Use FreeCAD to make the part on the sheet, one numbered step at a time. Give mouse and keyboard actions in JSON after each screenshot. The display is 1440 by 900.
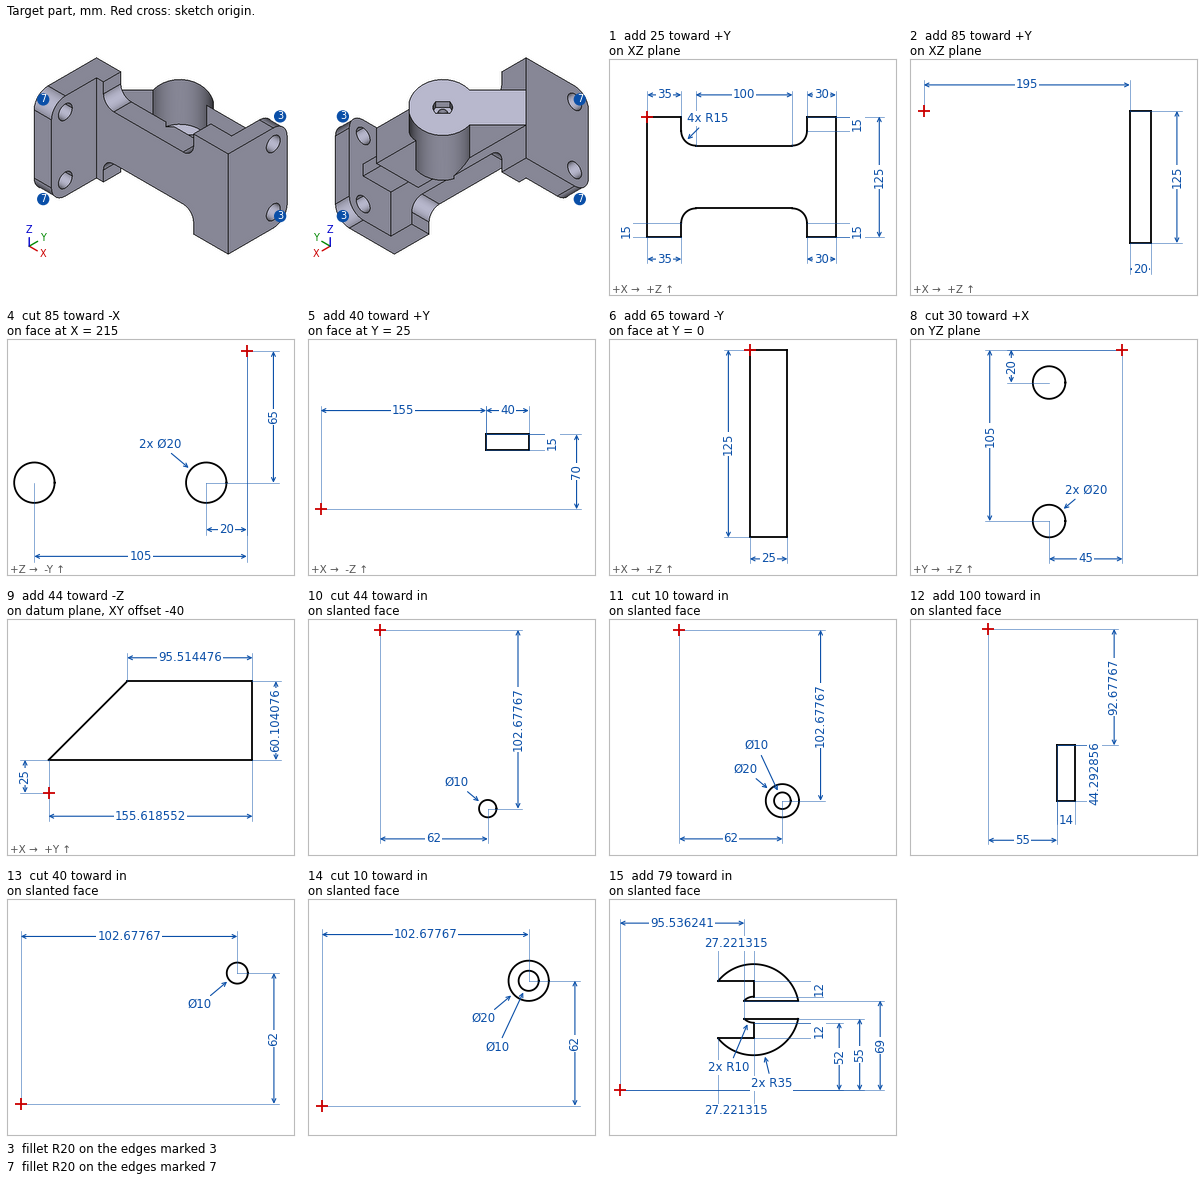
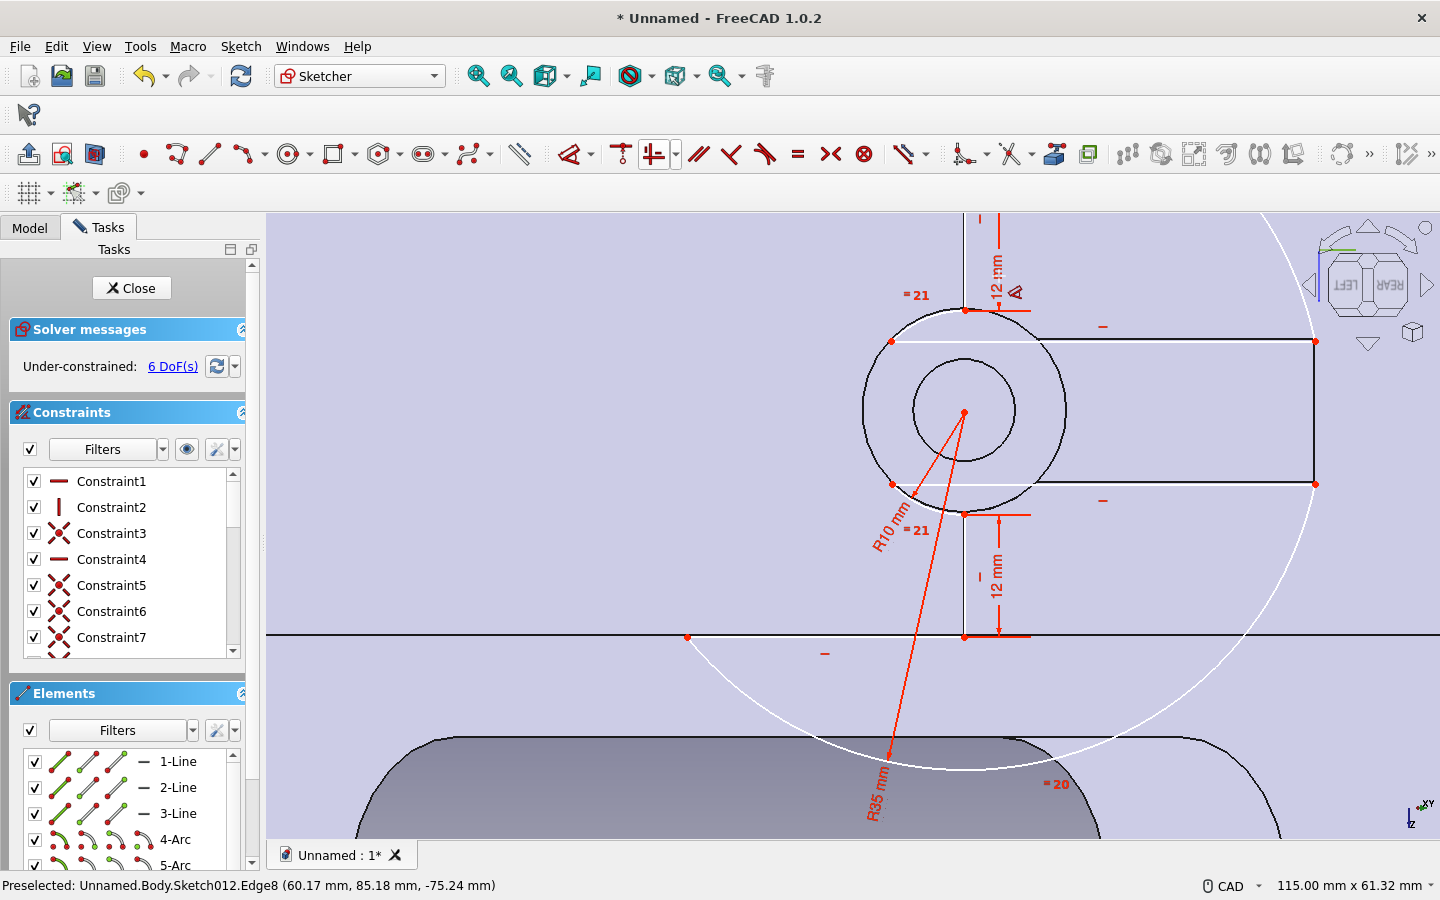
{"action": "scroll", "coordinate": [923, 504], "scroll_direction": "down", "scroll_amount": 4}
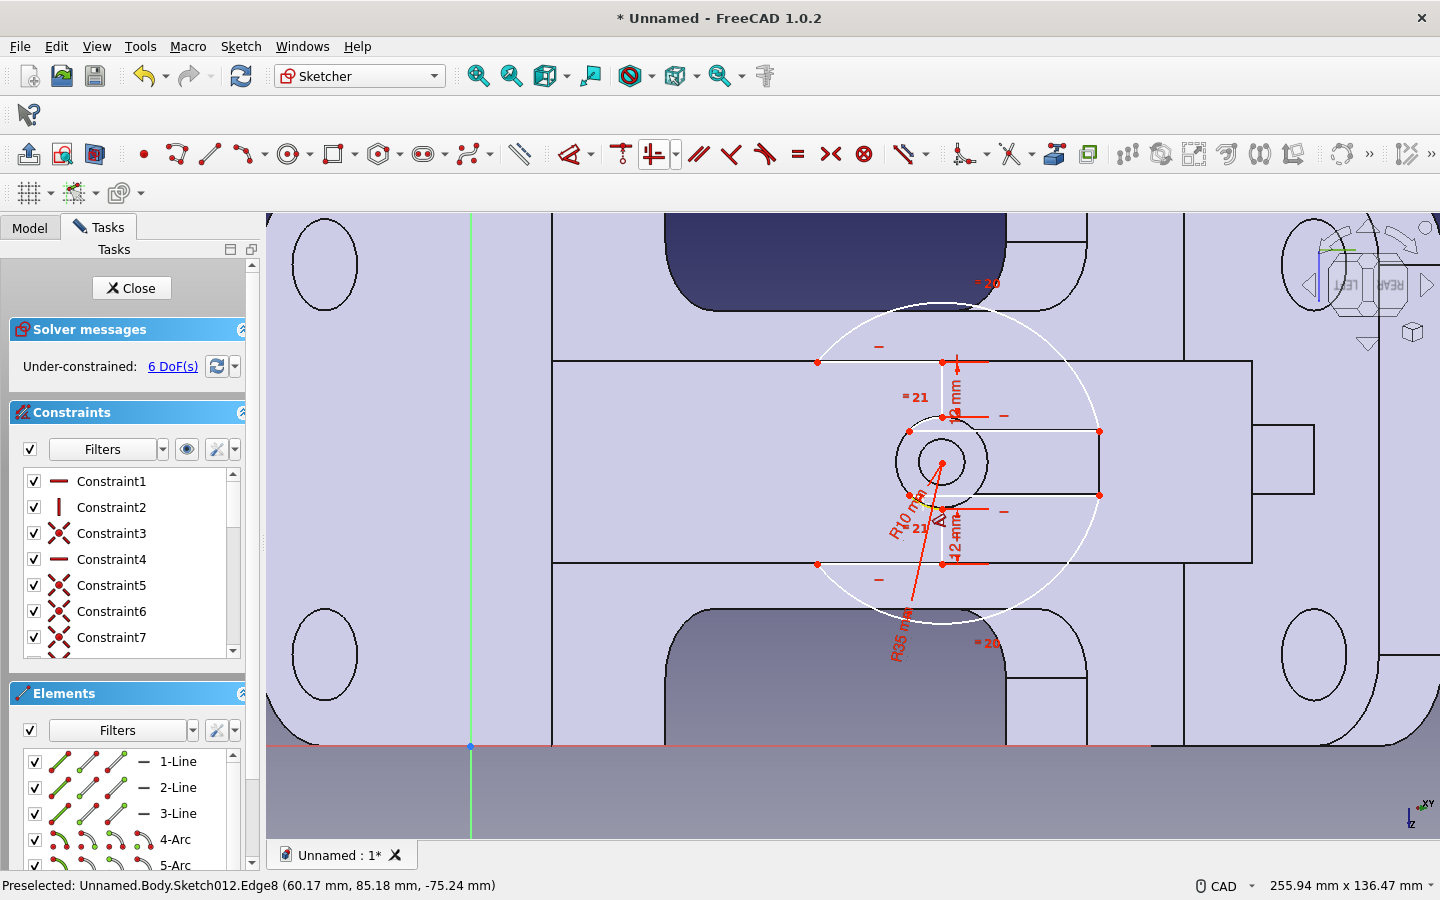
{"action": "left_click", "coordinate": [1099, 496]}
{"action": "left_click", "coordinate": [1133, 621]}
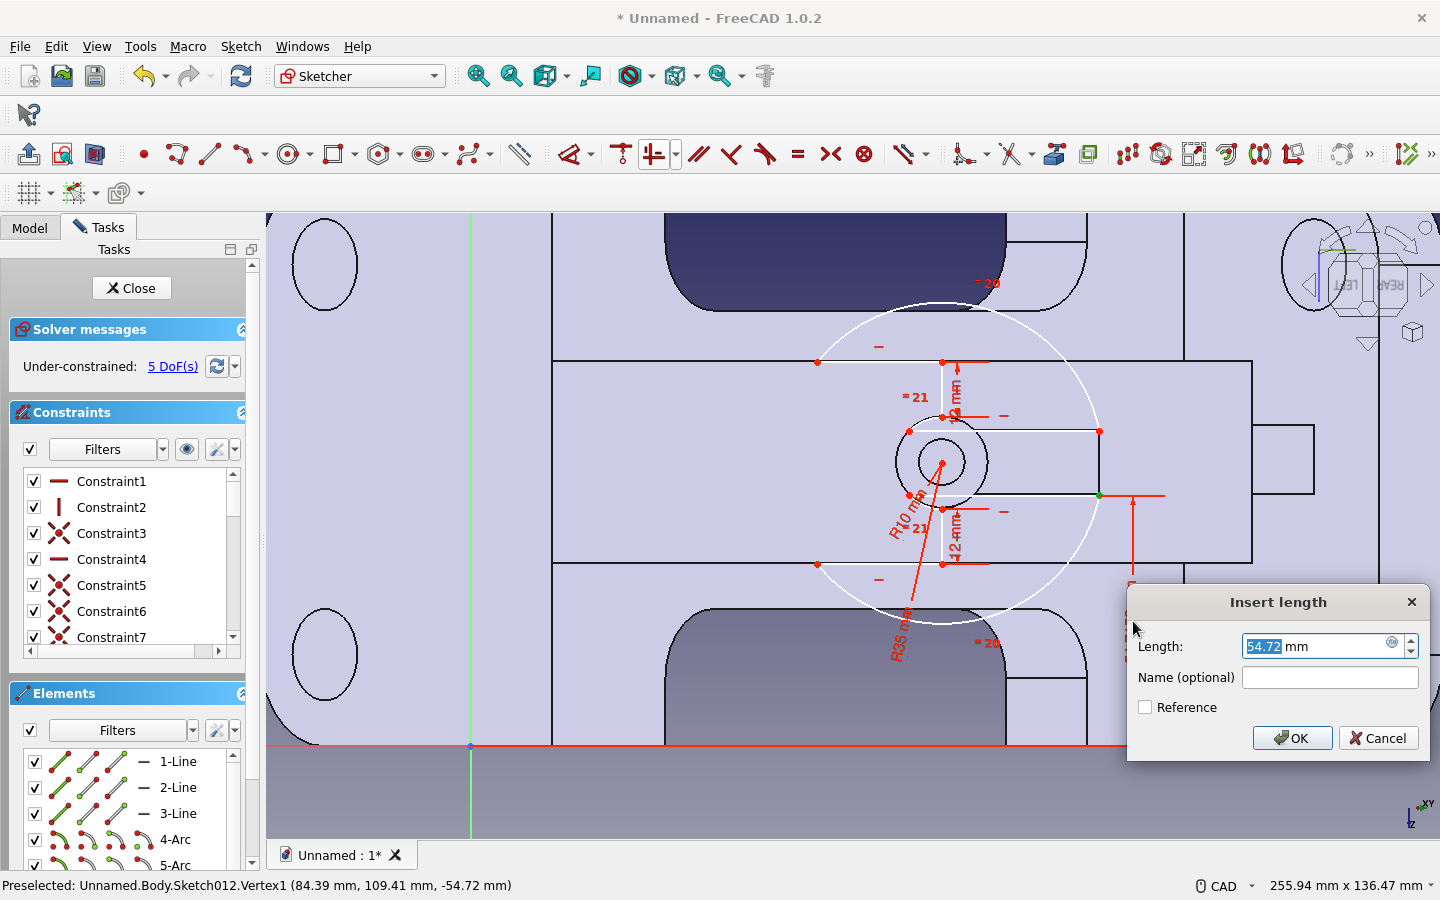
{"action": "type", "text": "55"}
{"action": "key", "text": "Return"}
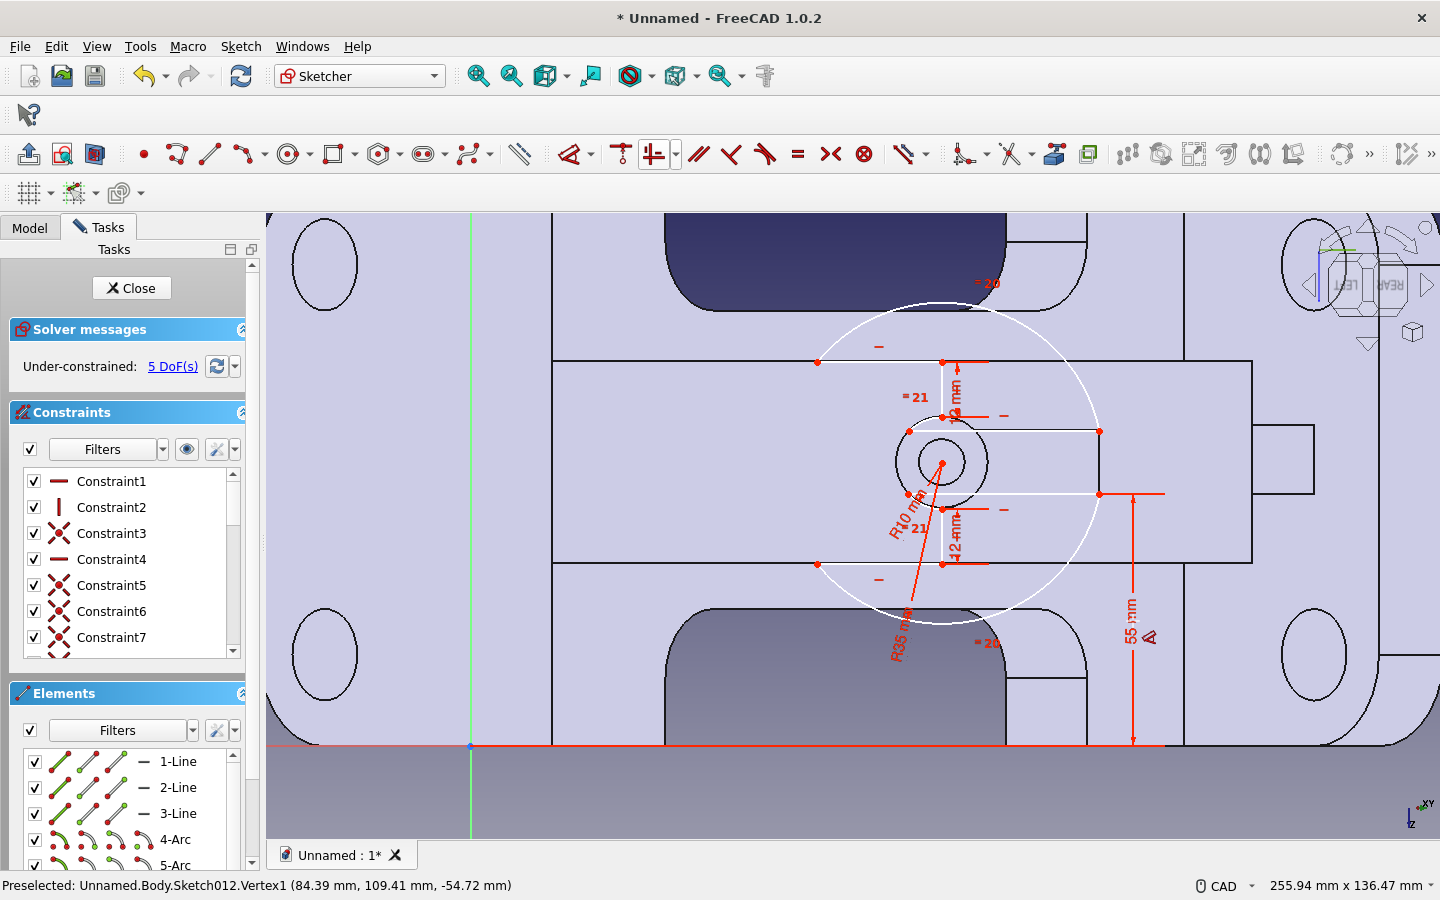
{"action": "left_click", "coordinate": [942, 509]}
{"action": "left_click", "coordinate": [437, 628]}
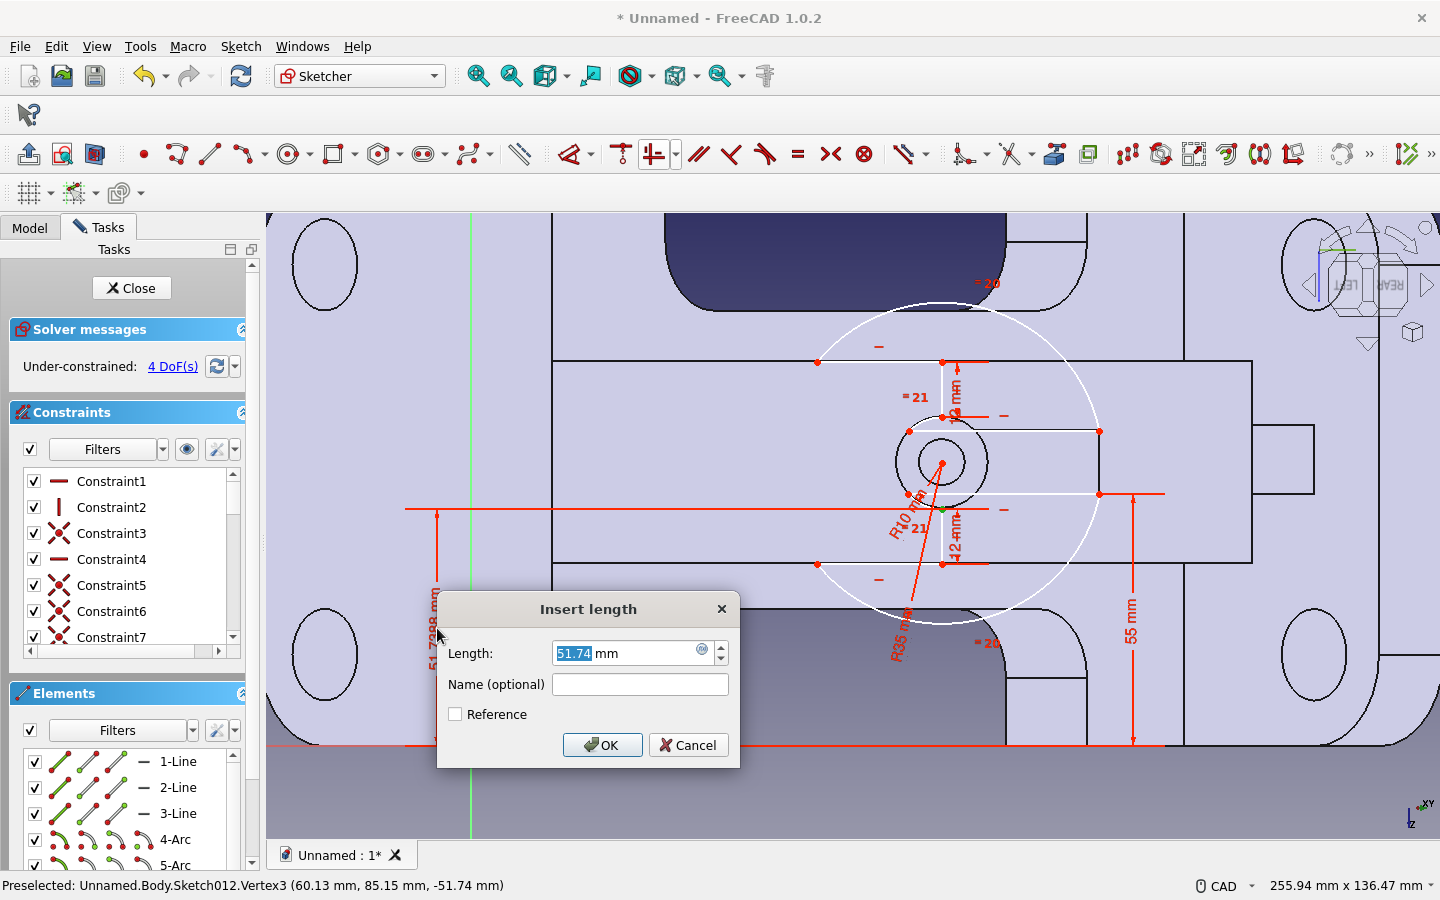
{"action": "type", "text": "52"}
{"action": "key", "text": "Return"}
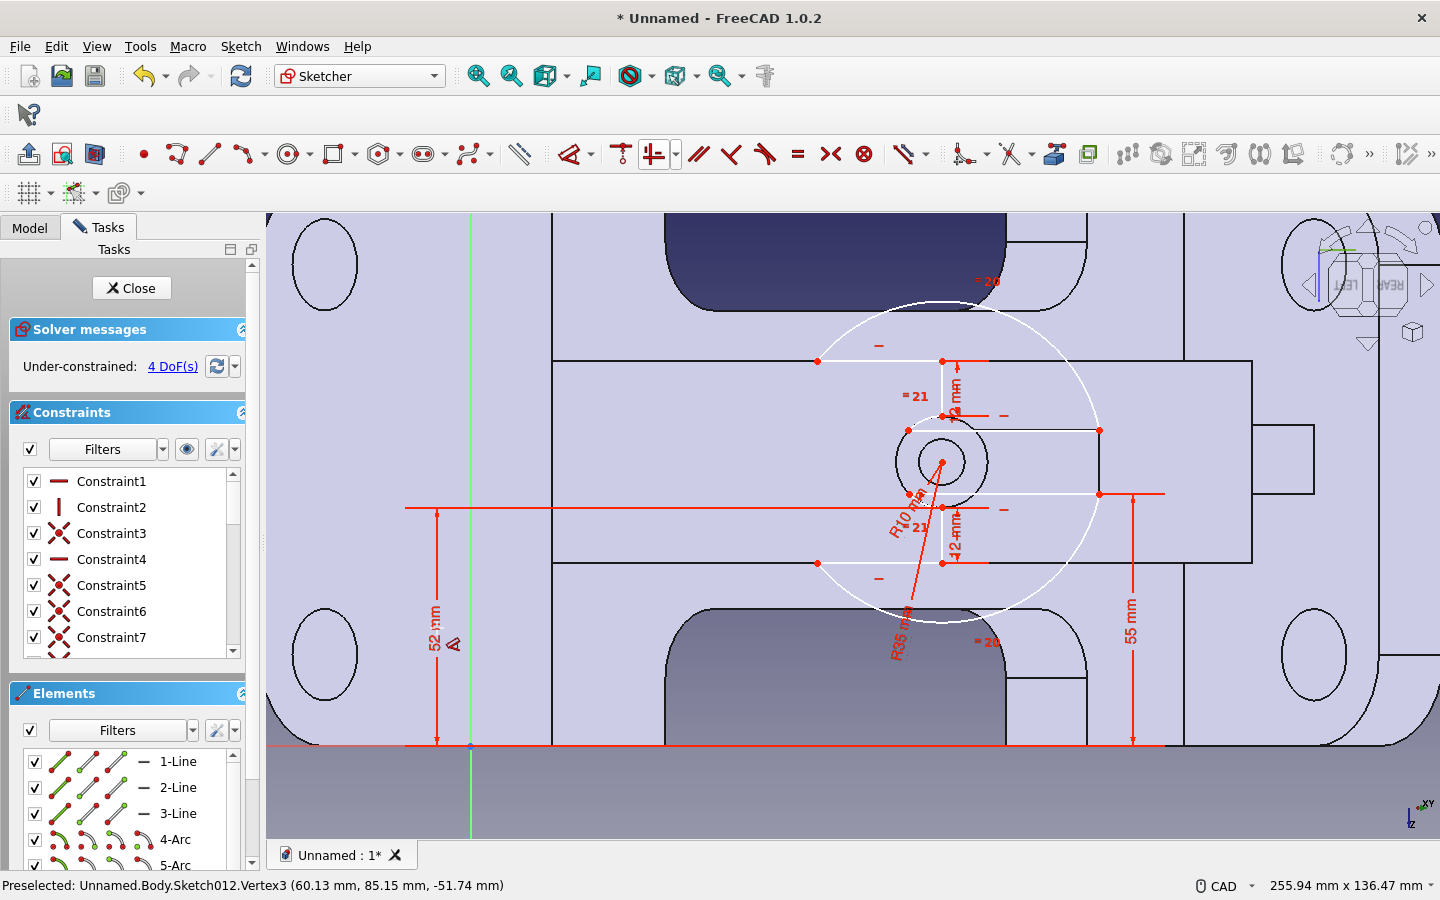
{"action": "left_click", "coordinate": [909, 431]}
{"action": "left_click", "coordinate": [437, 589]}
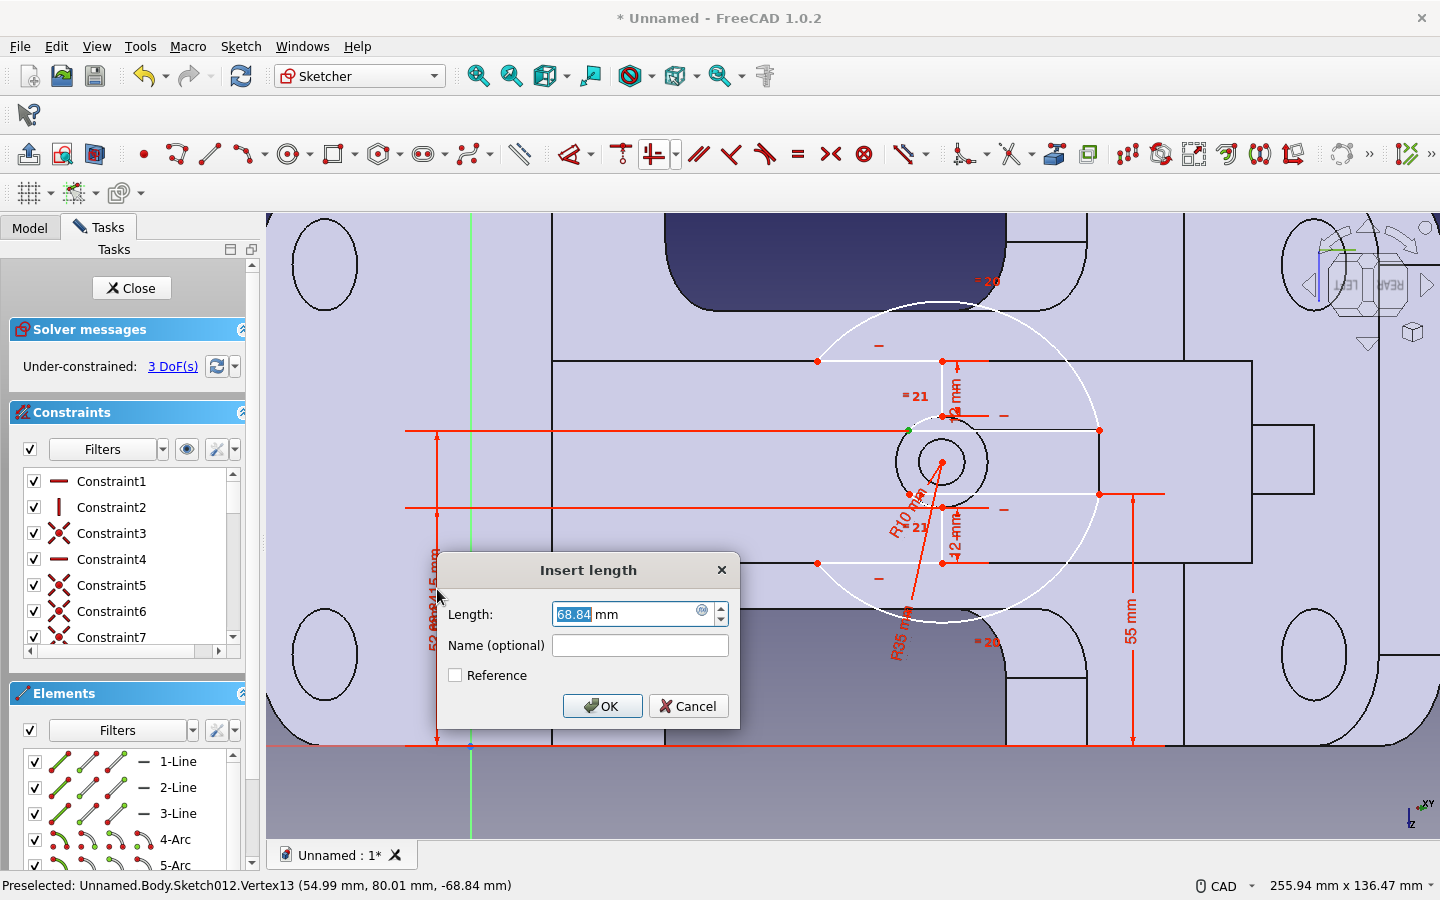
{"action": "type", "text": "69"}
{"action": "key", "text": "Return"}